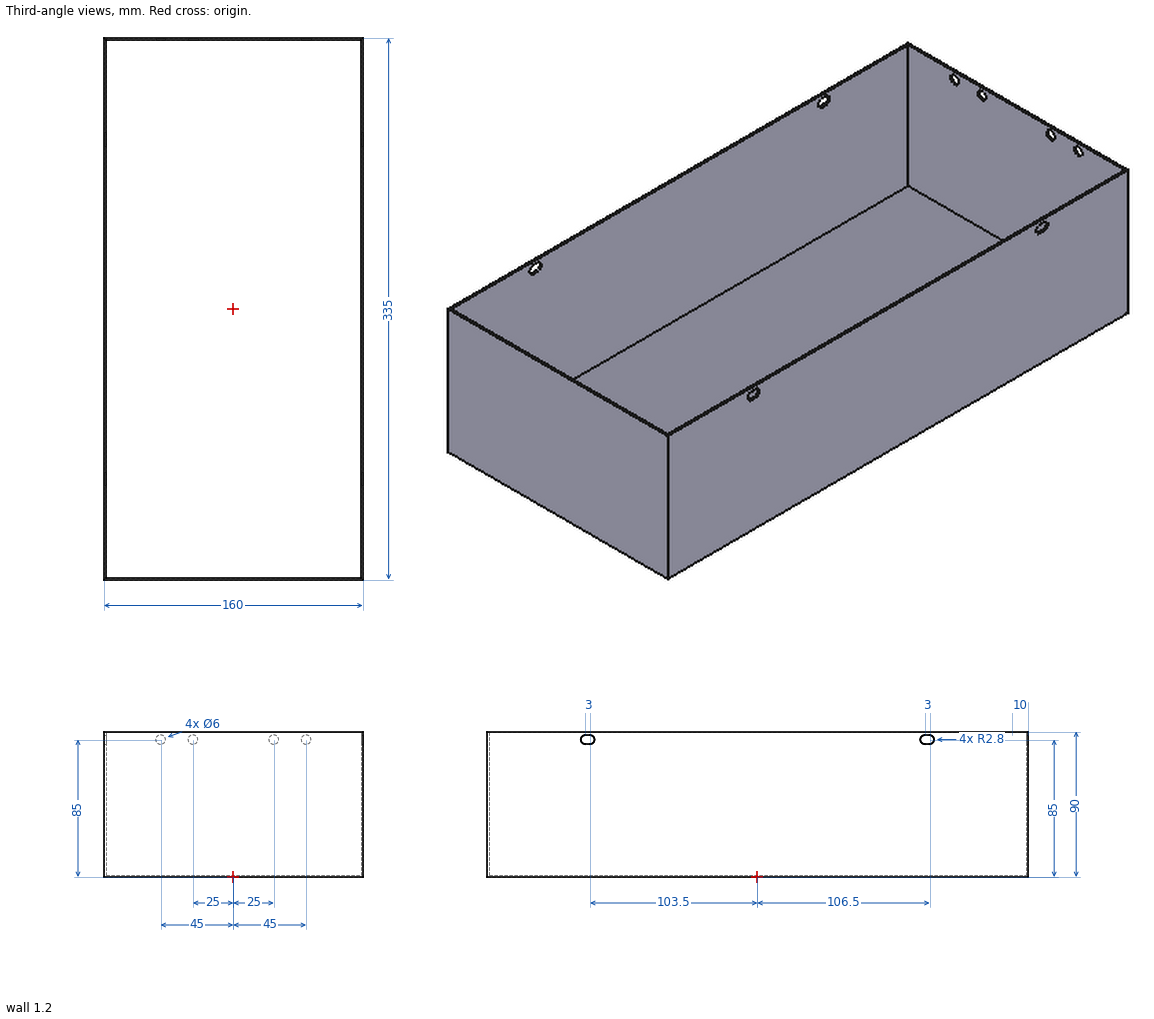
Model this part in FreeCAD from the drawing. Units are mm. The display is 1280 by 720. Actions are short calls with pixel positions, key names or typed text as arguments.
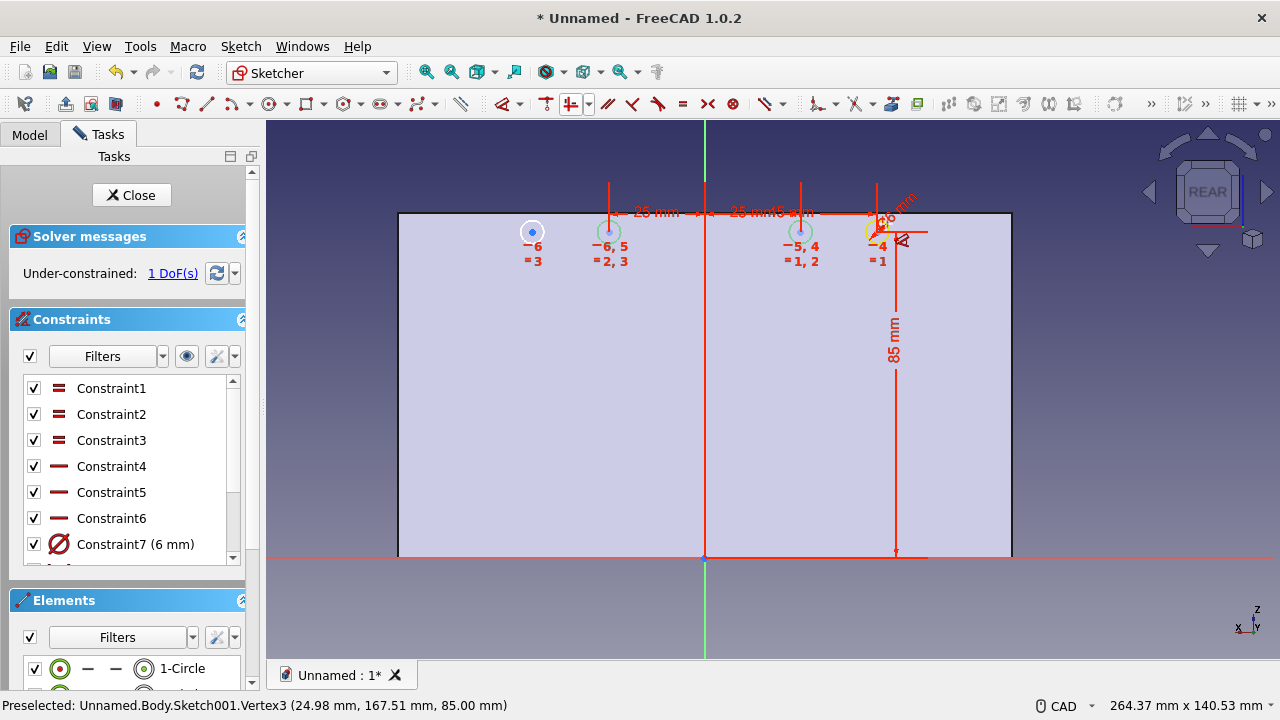
click(532, 232)
click(619, 592)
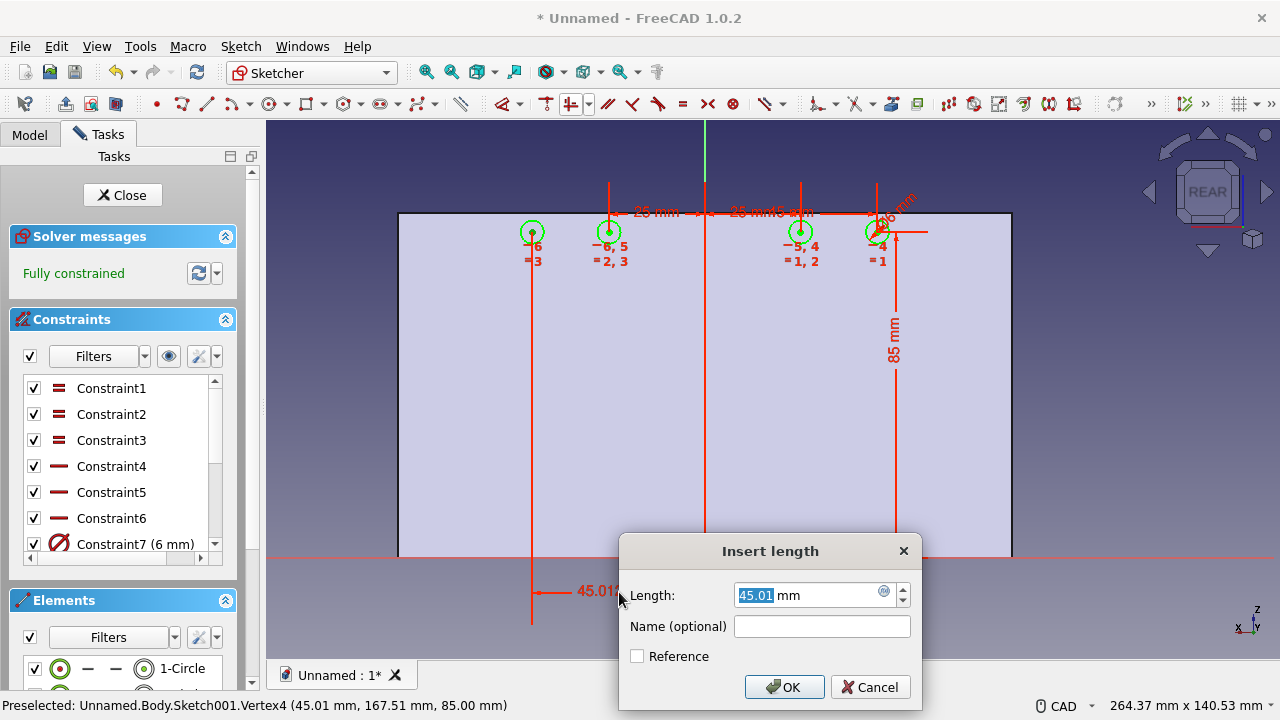
text(45)
key(Return)
key(Escape)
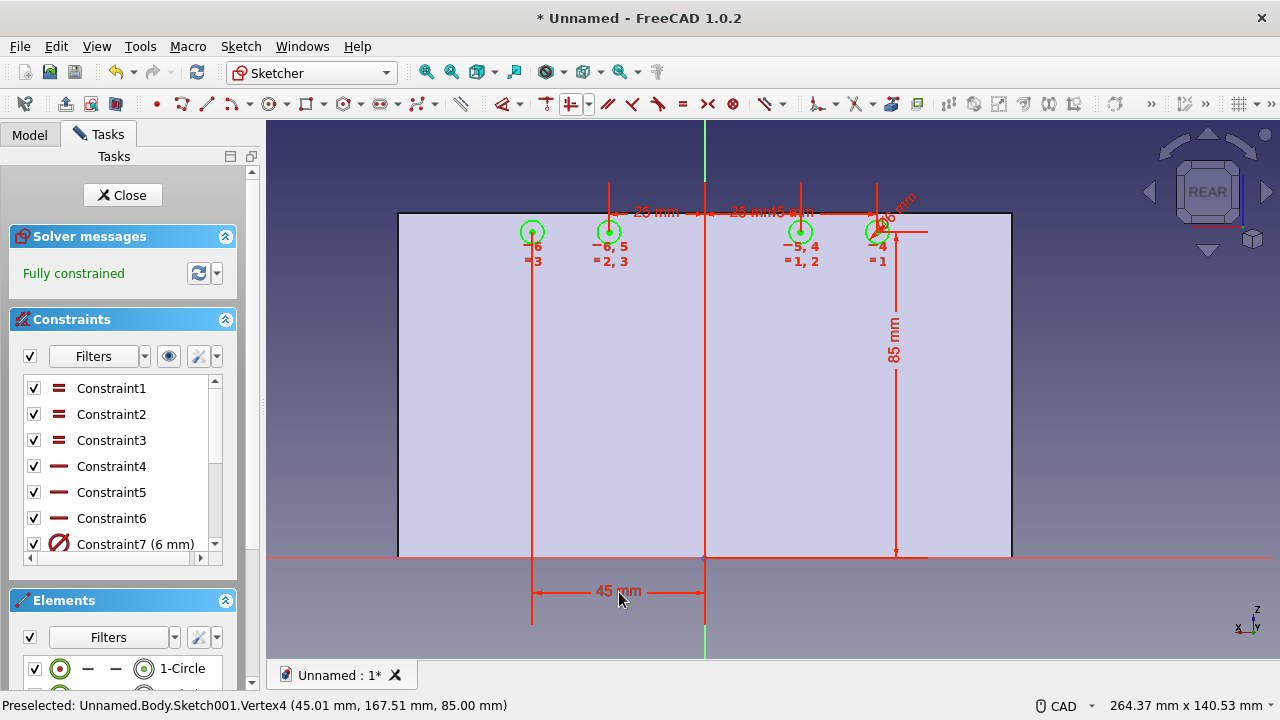
click(123, 195)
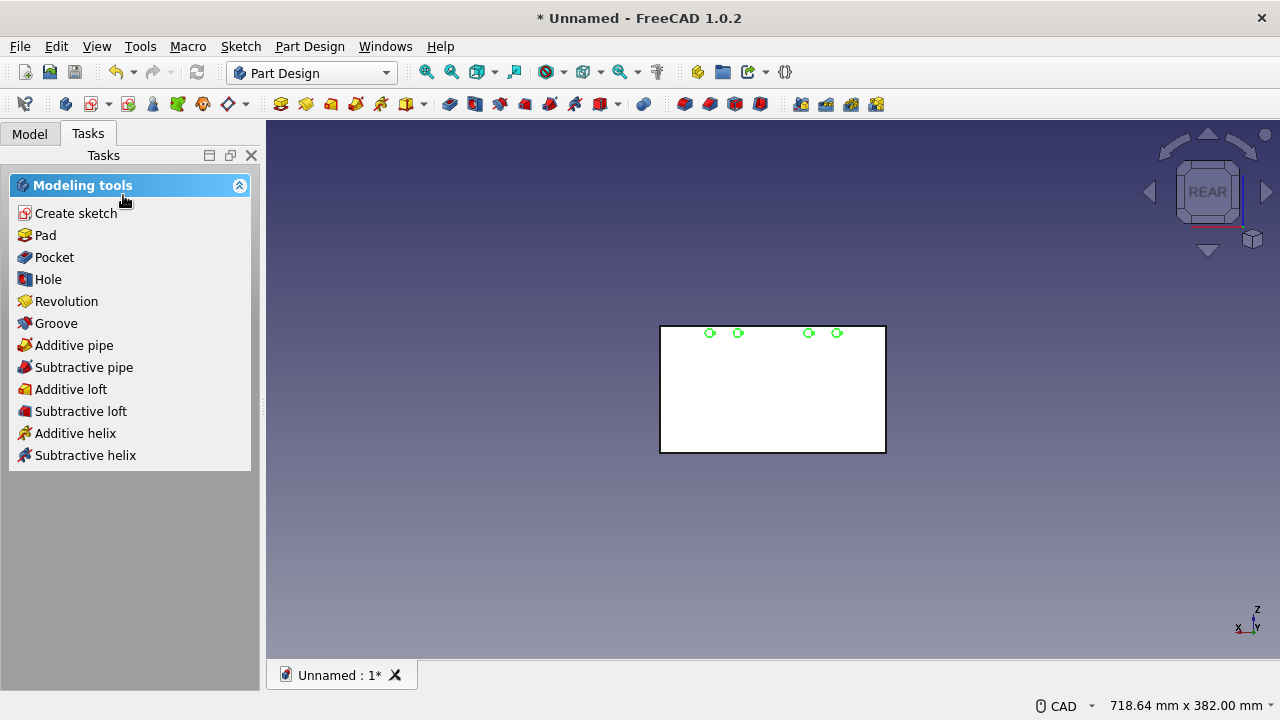
click(450, 104)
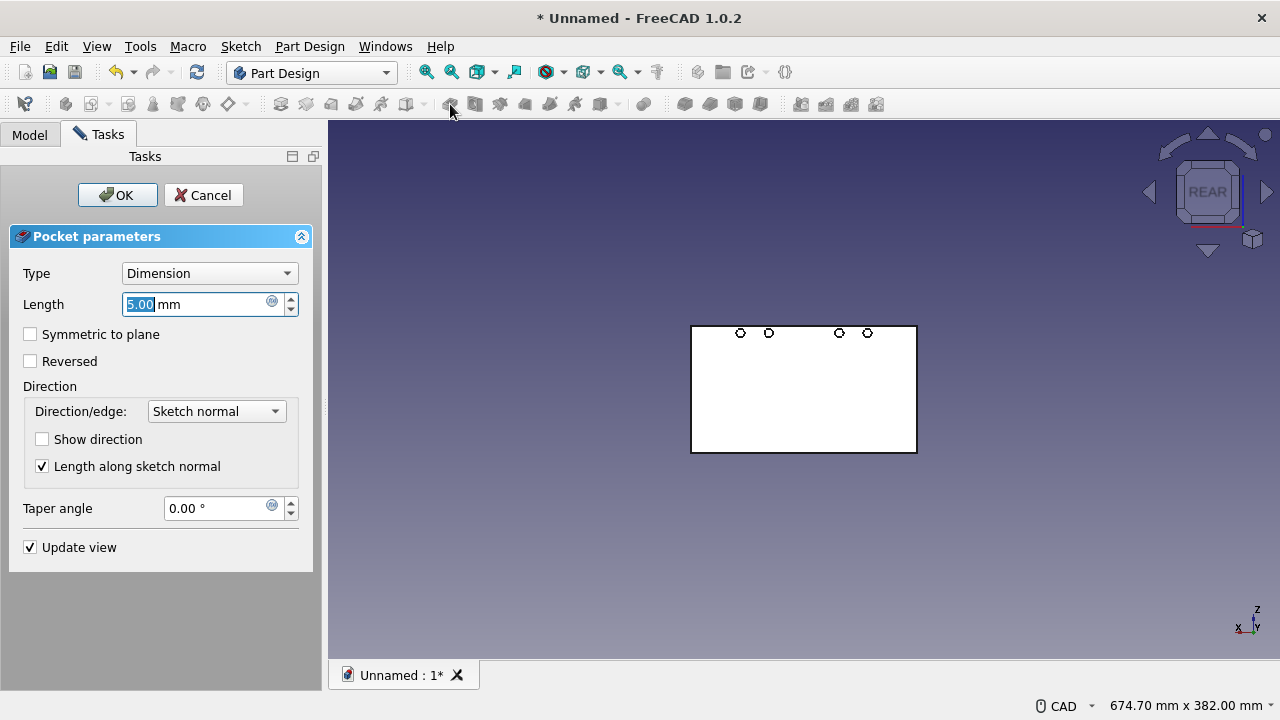
text(10)
key(Tab)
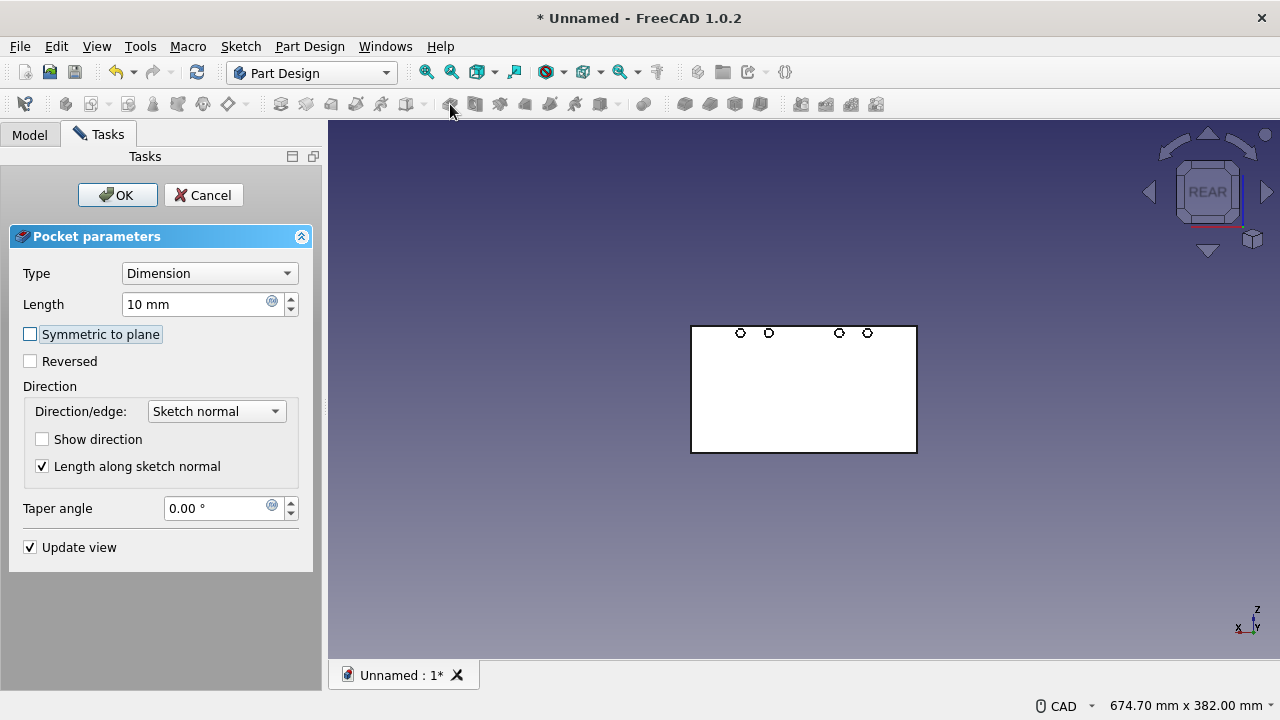
click(118, 195)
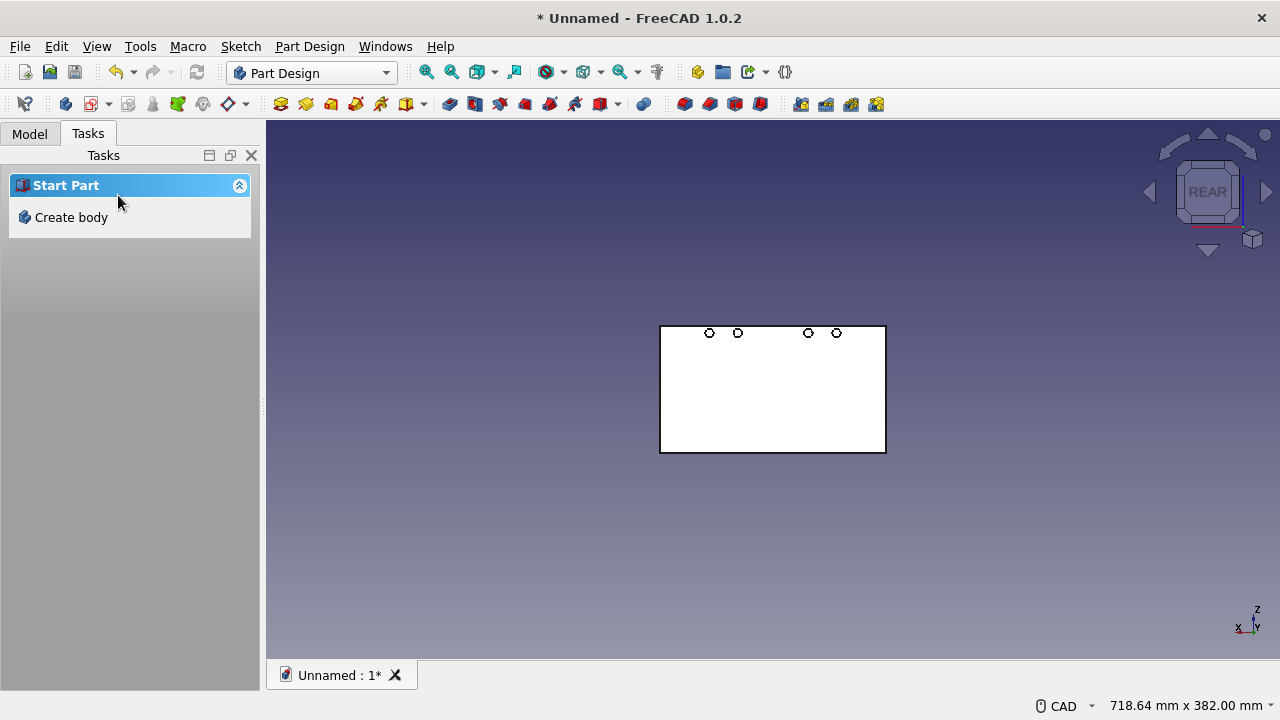
key(v)
key(f)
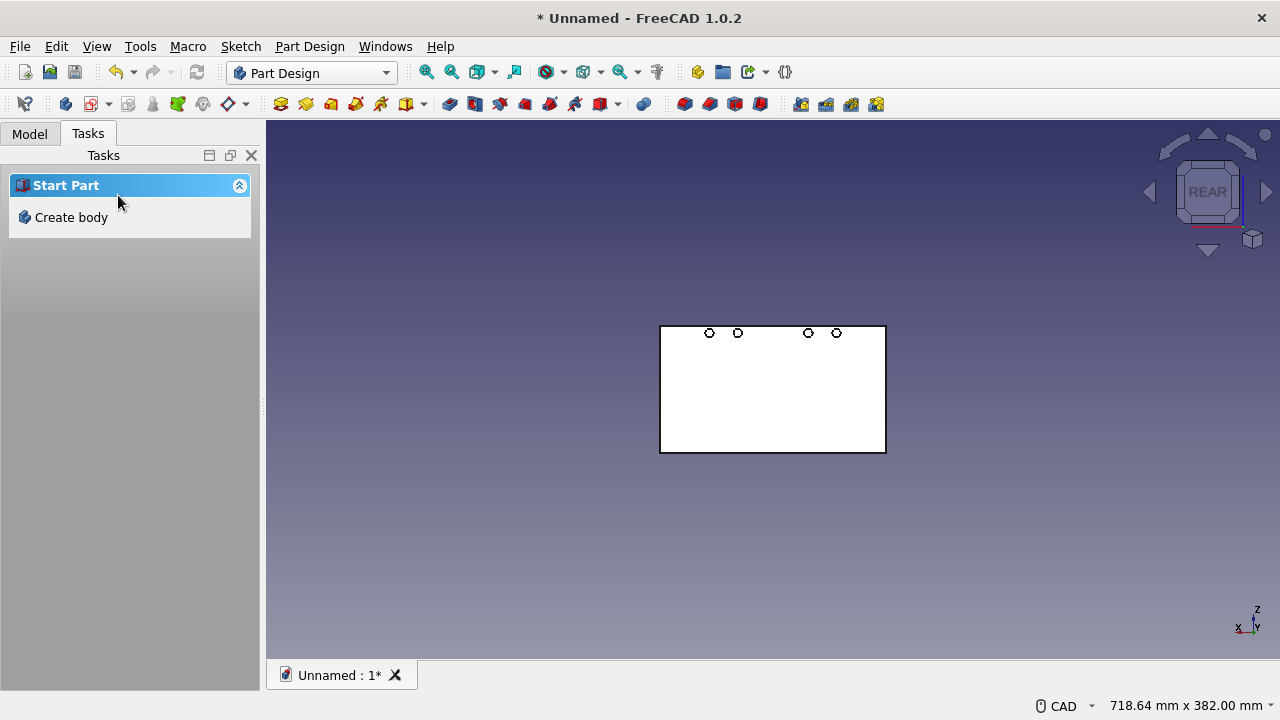
key(6)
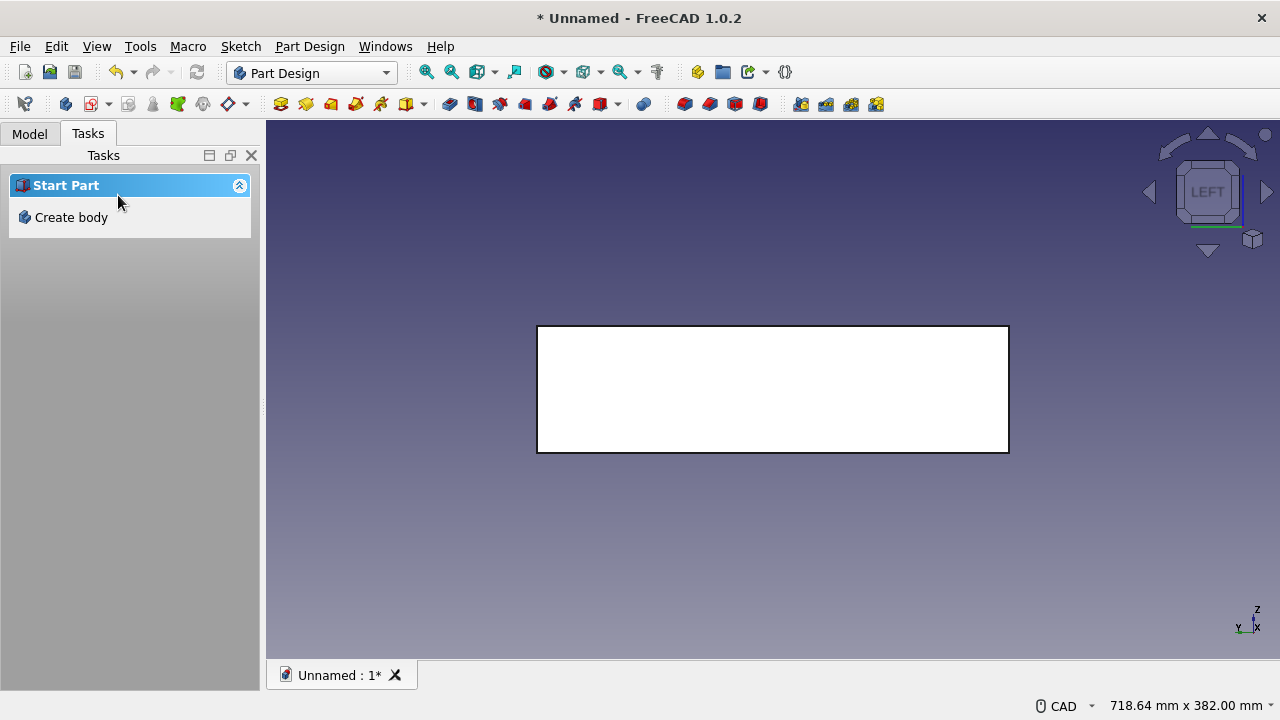
click(638, 388)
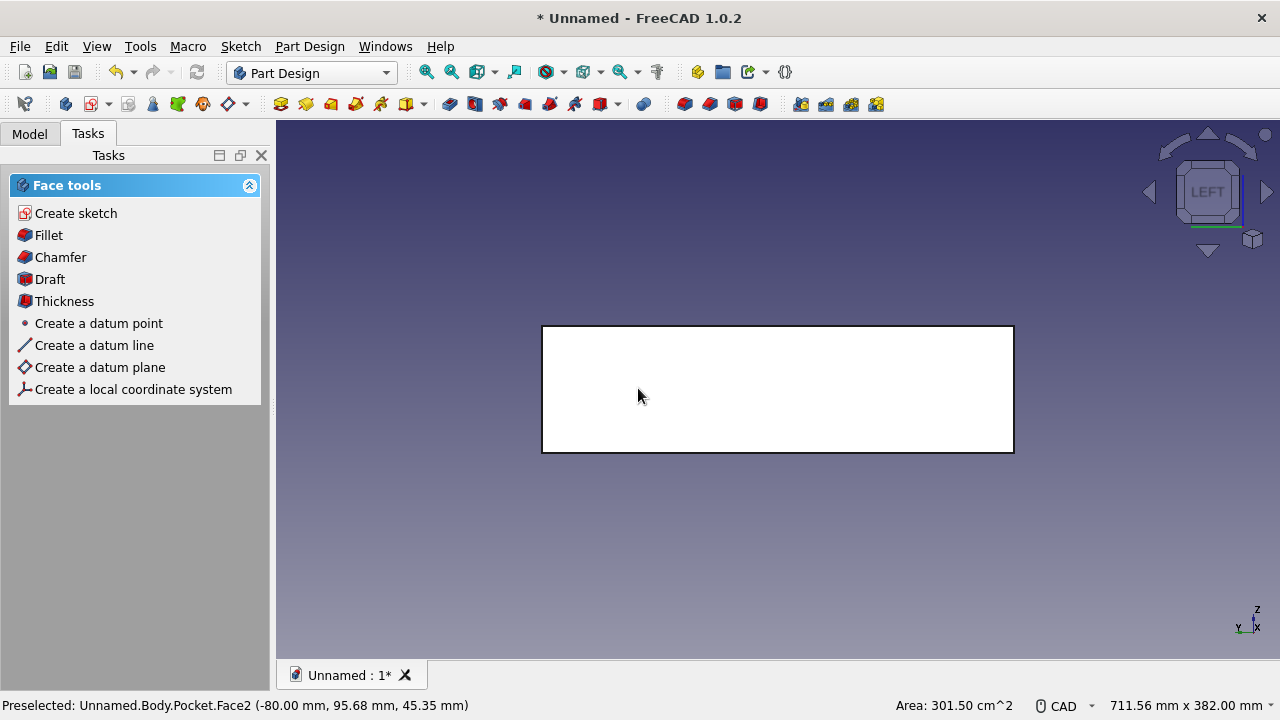
click(90, 104)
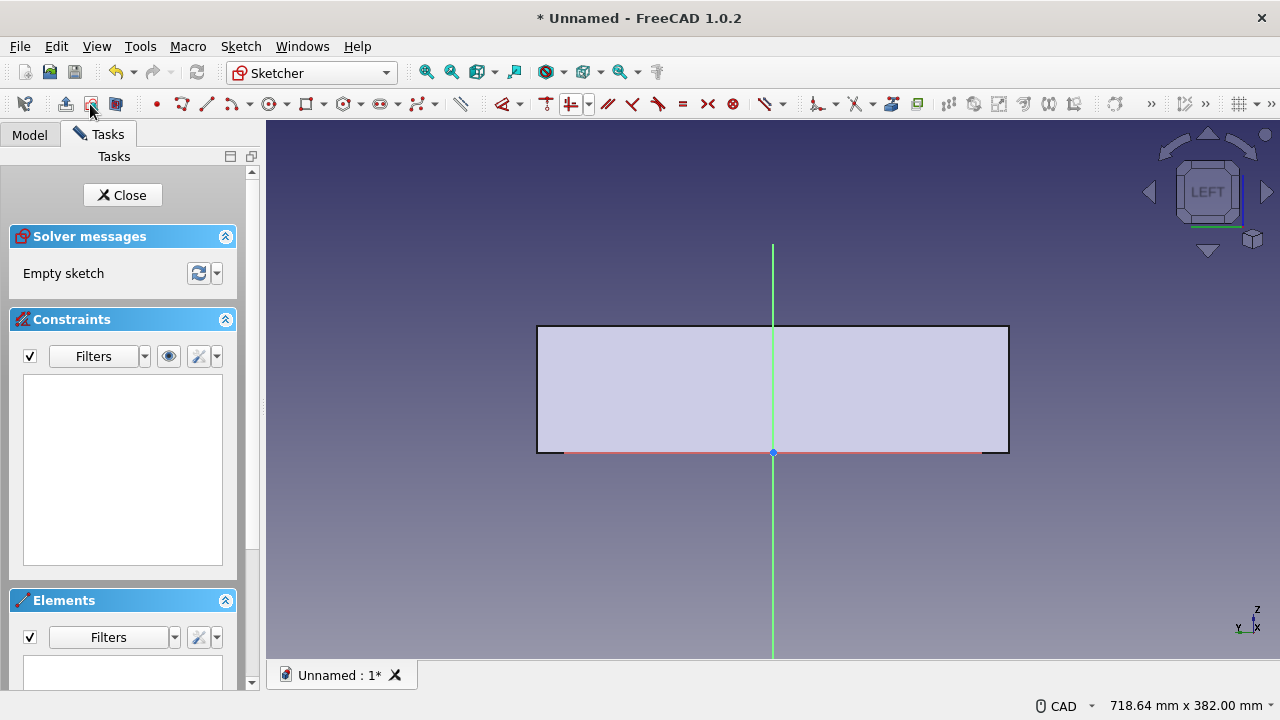
scroll(856, 393, up, 3)